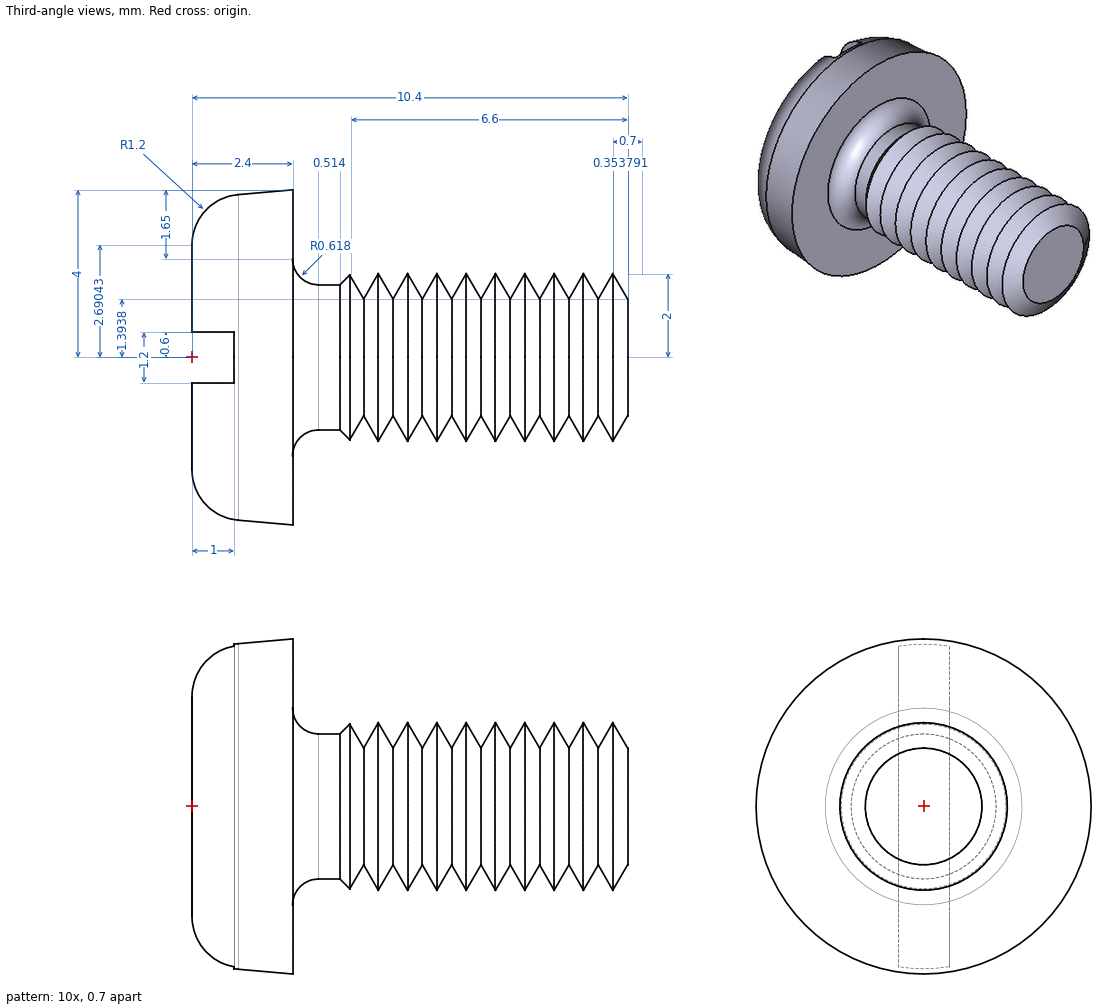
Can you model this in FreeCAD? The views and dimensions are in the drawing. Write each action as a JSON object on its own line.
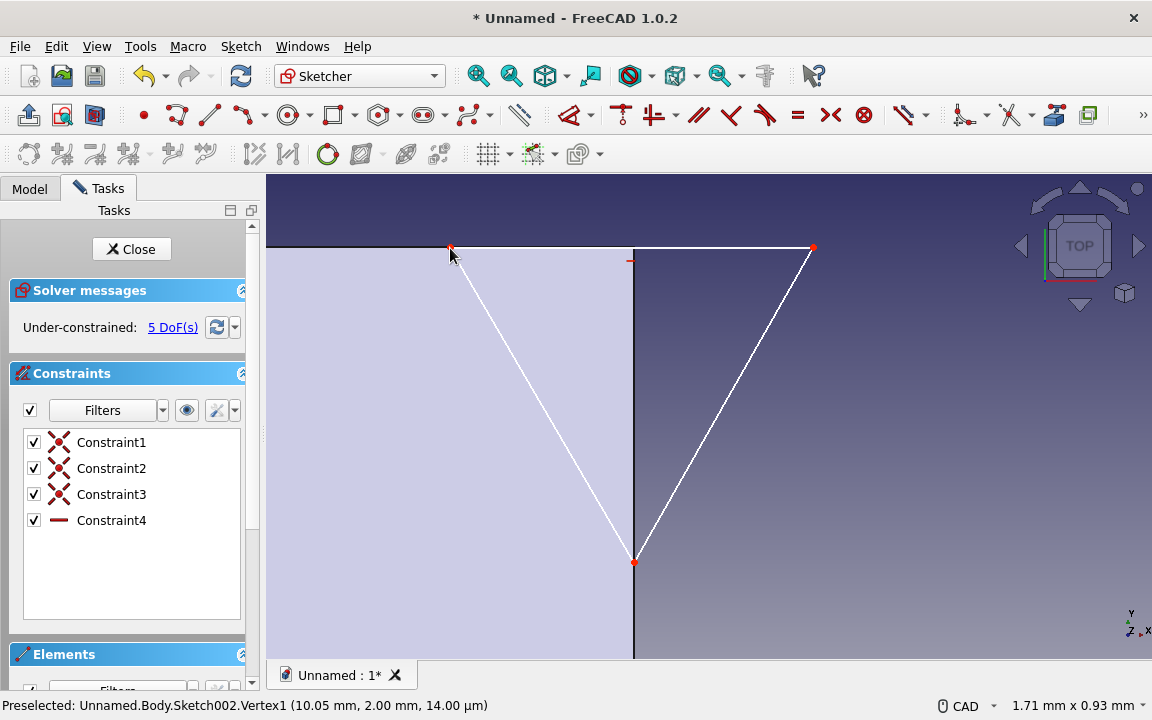
{"action": "left_click", "coordinate": [568, 116]}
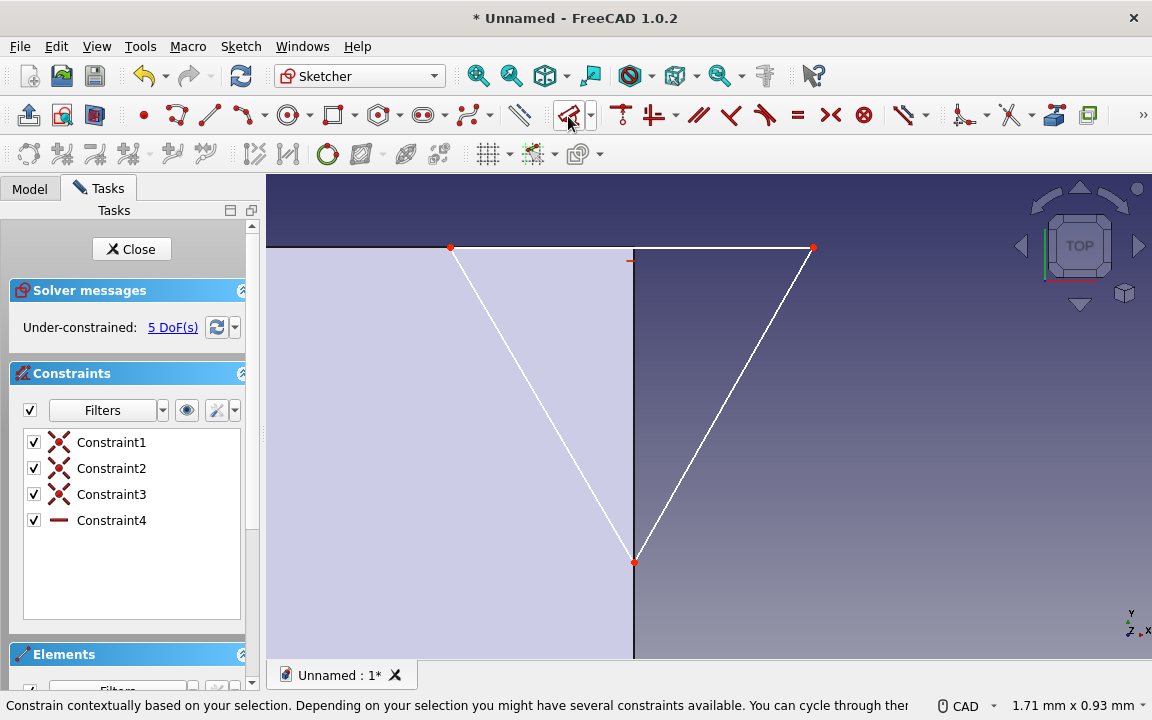
{"action": "left_click", "coordinate": [450, 248]}
{"action": "left_click", "coordinate": [484, 440]}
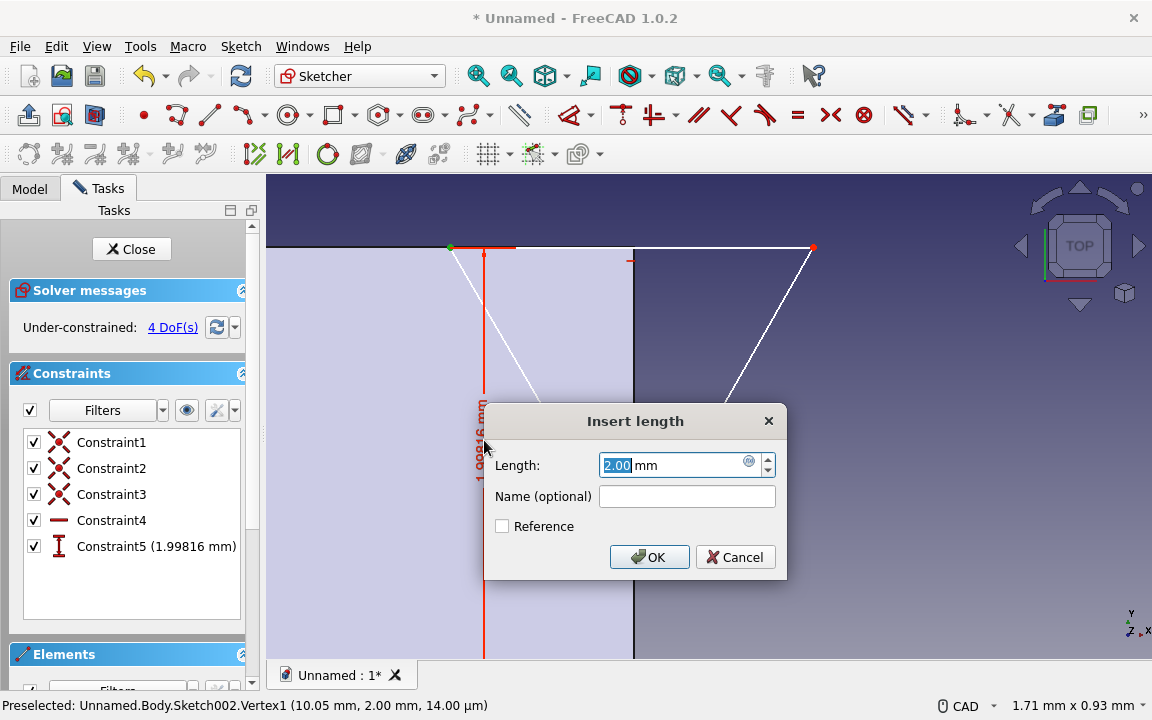
{"action": "type", "text": "2"}
{"action": "key", "text": "Return"}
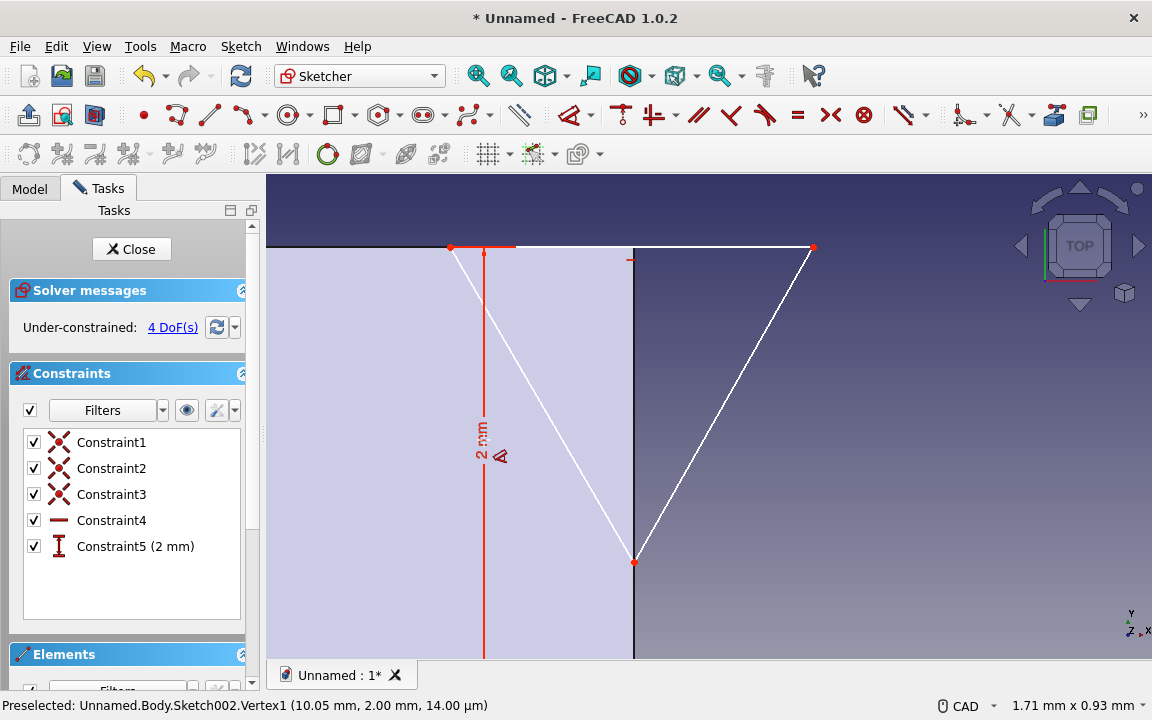
{"action": "left_click", "coordinate": [704, 247]}
{"action": "left_click", "coordinate": [632, 213]}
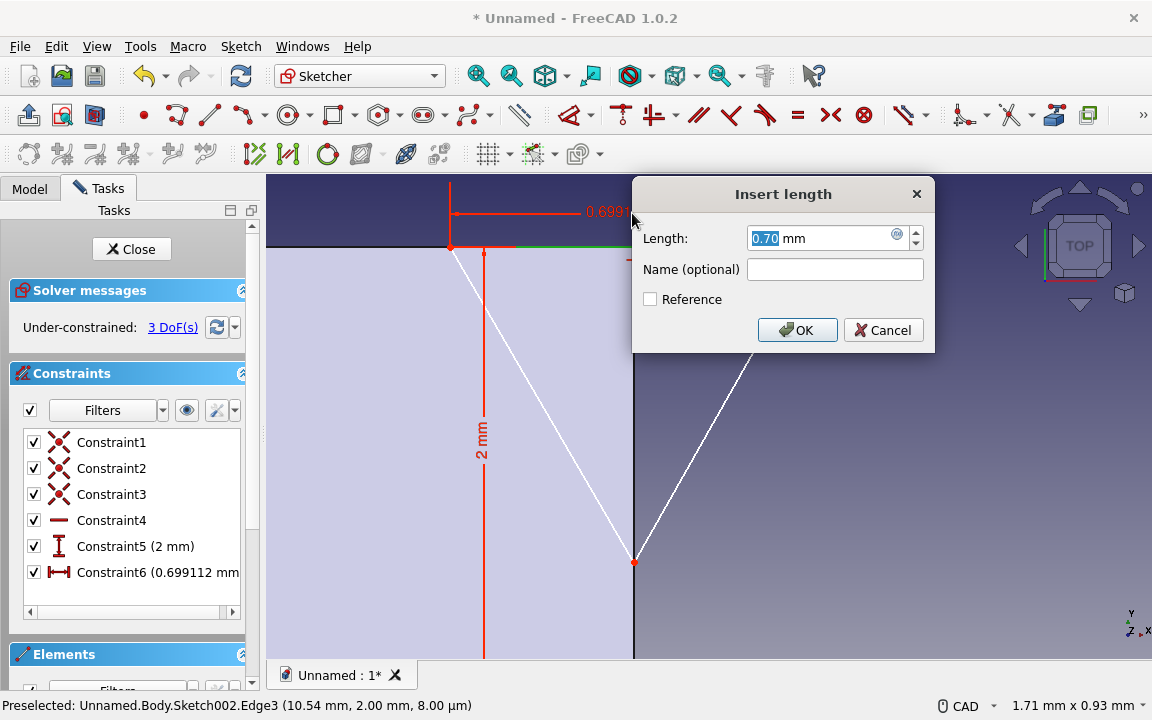
{"action": "type", "text": "0.7"}
{"action": "key", "text": "Return"}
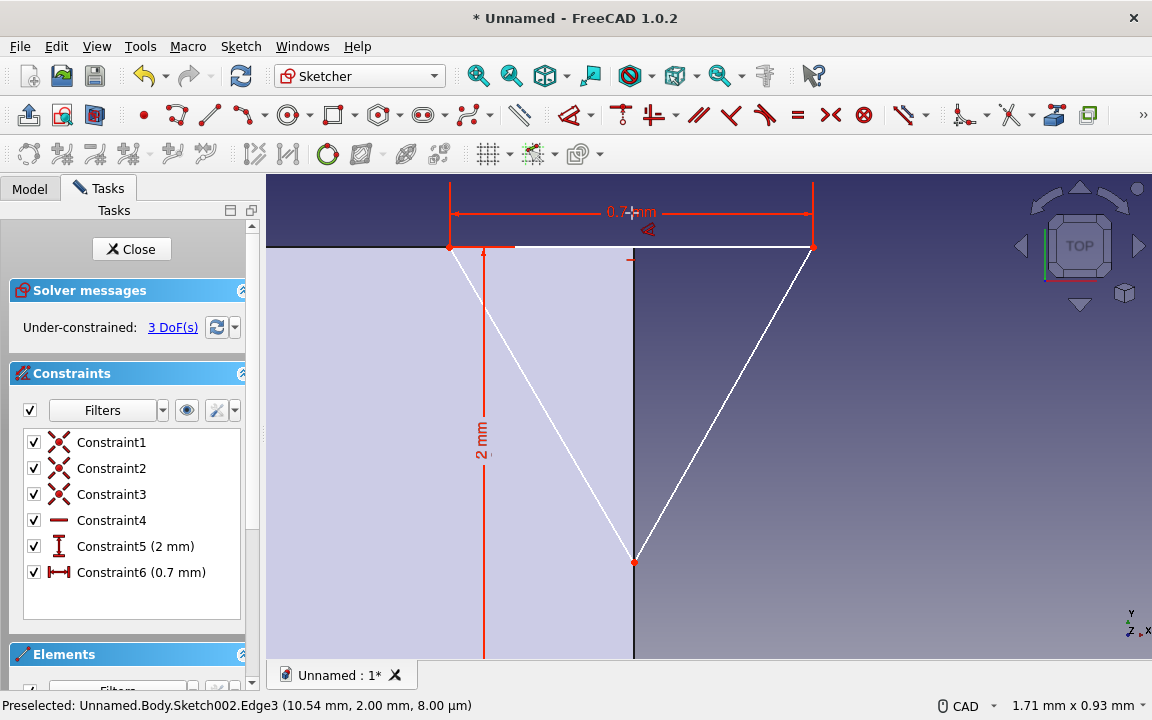
{"action": "left_click", "coordinate": [634, 563]}
{"action": "left_click", "coordinate": [464, 529]}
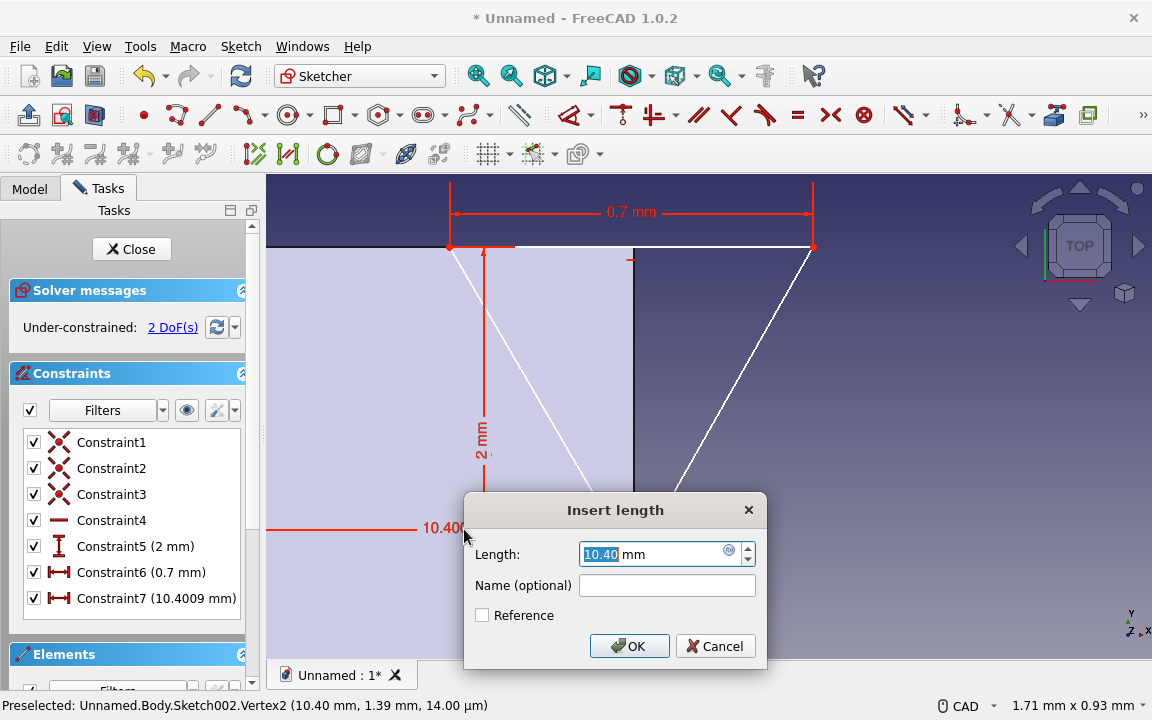
{"action": "type", "text": "10.4"}
{"action": "key", "text": "Return"}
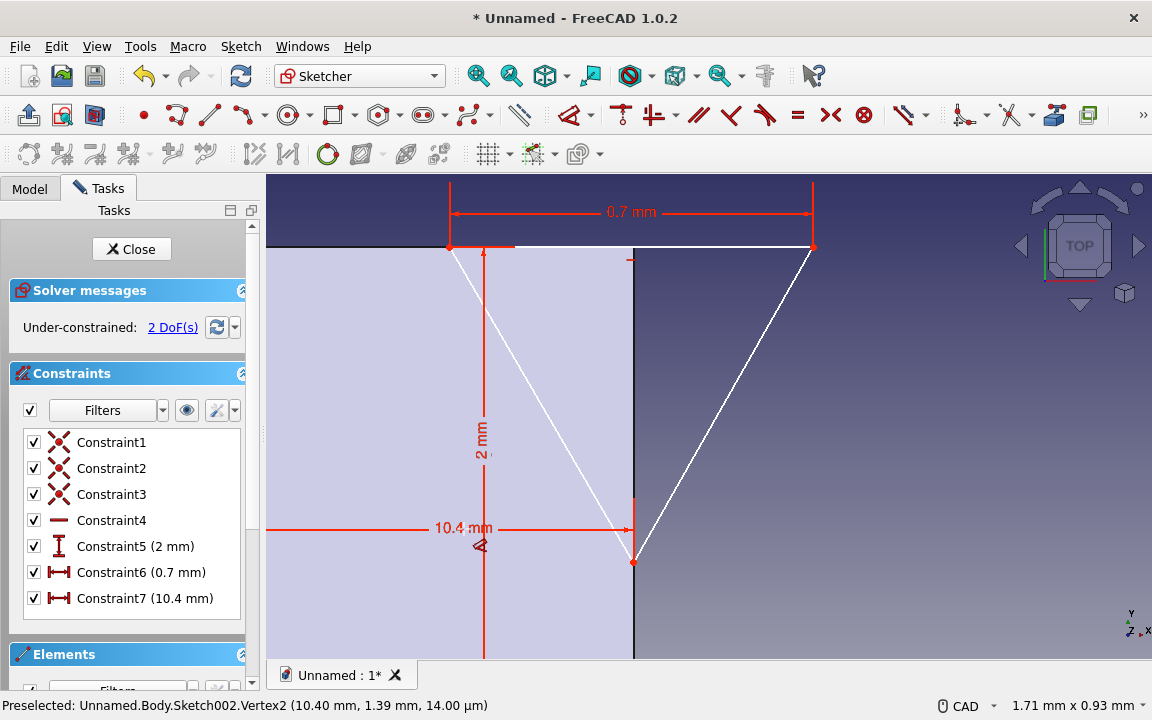
{"action": "left_click", "coordinate": [634, 563]}
{"action": "left_click", "coordinate": [668, 597]}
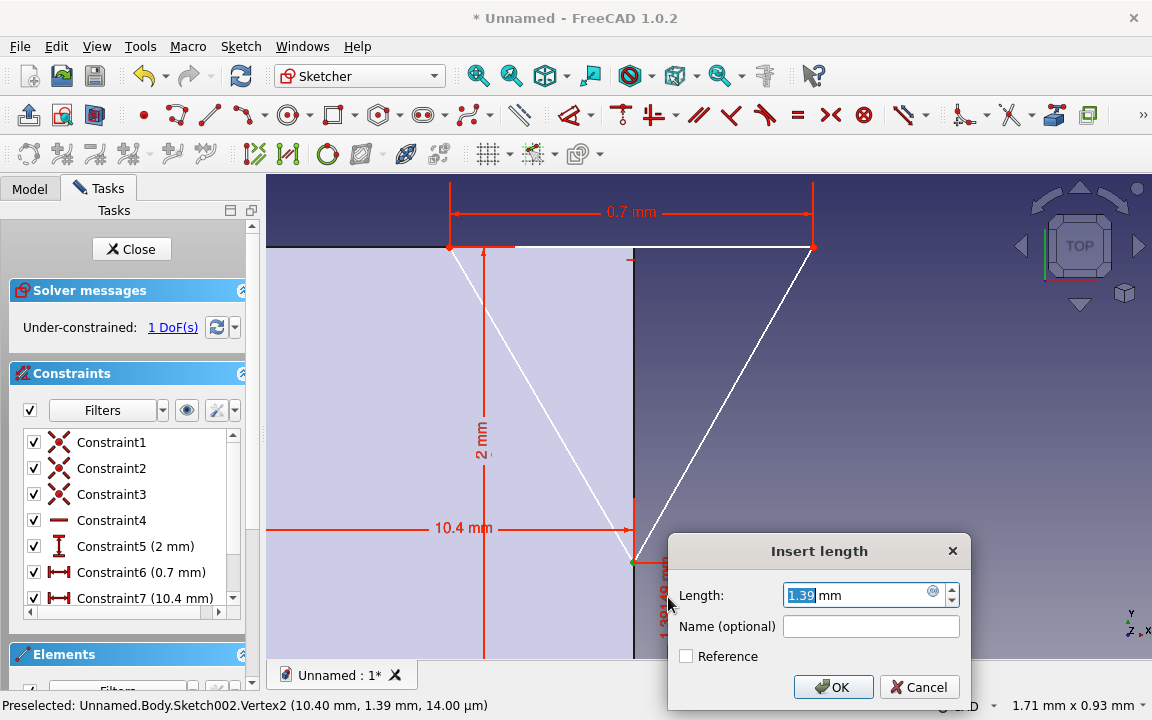
{"action": "type", "text": "1.3938"}
{"action": "key", "text": "Return"}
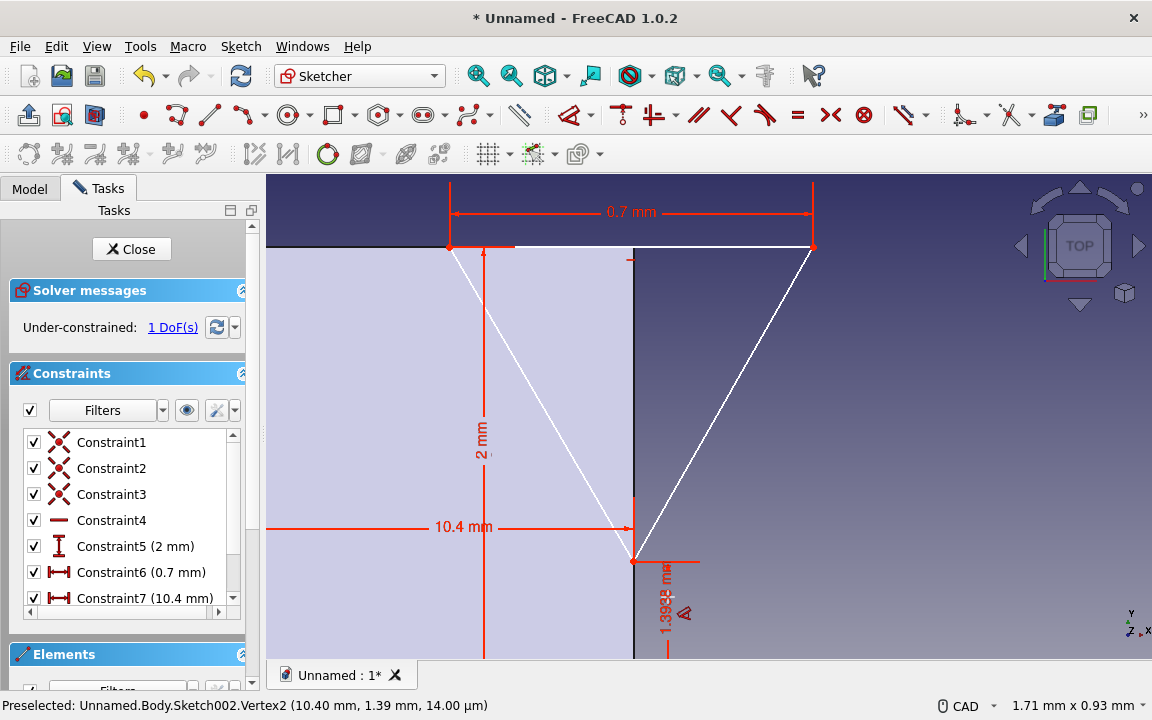
{"action": "left_click", "coordinate": [505, 341]}
{"action": "left_click", "coordinate": [542, 596]}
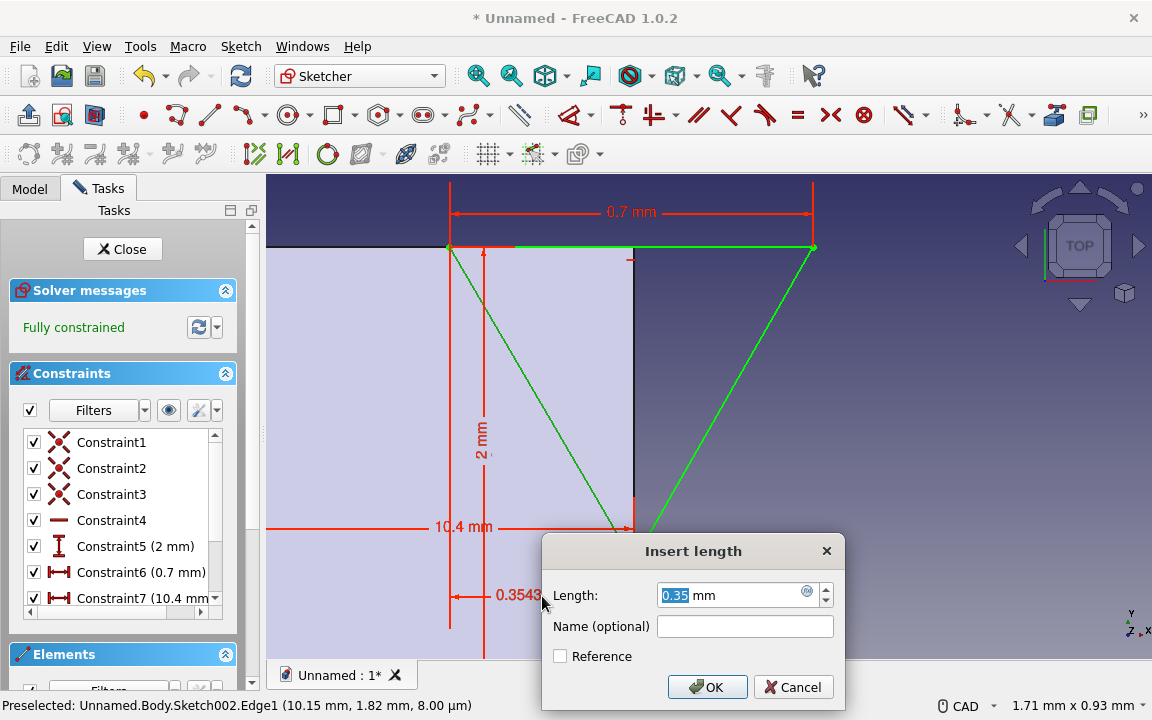
{"action": "type", "text": "0.353791"}
{"action": "key", "text": "Return"}
{"action": "key", "text": "Escape"}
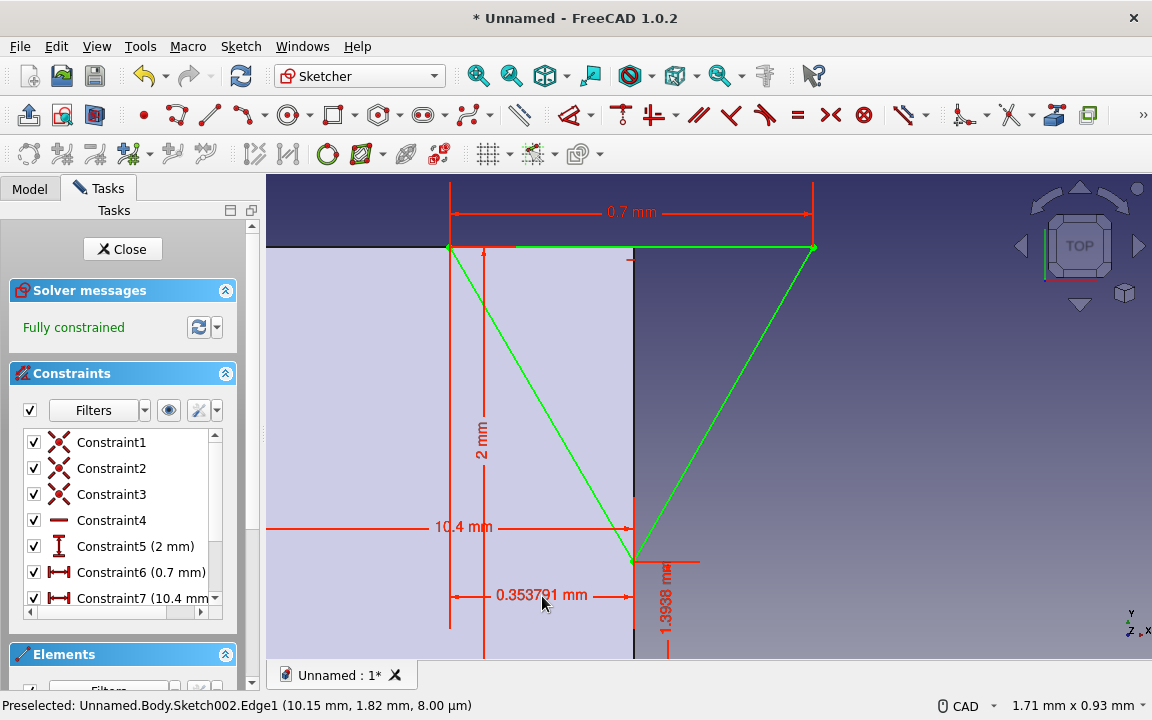
{"action": "left_click", "coordinate": [123, 249]}